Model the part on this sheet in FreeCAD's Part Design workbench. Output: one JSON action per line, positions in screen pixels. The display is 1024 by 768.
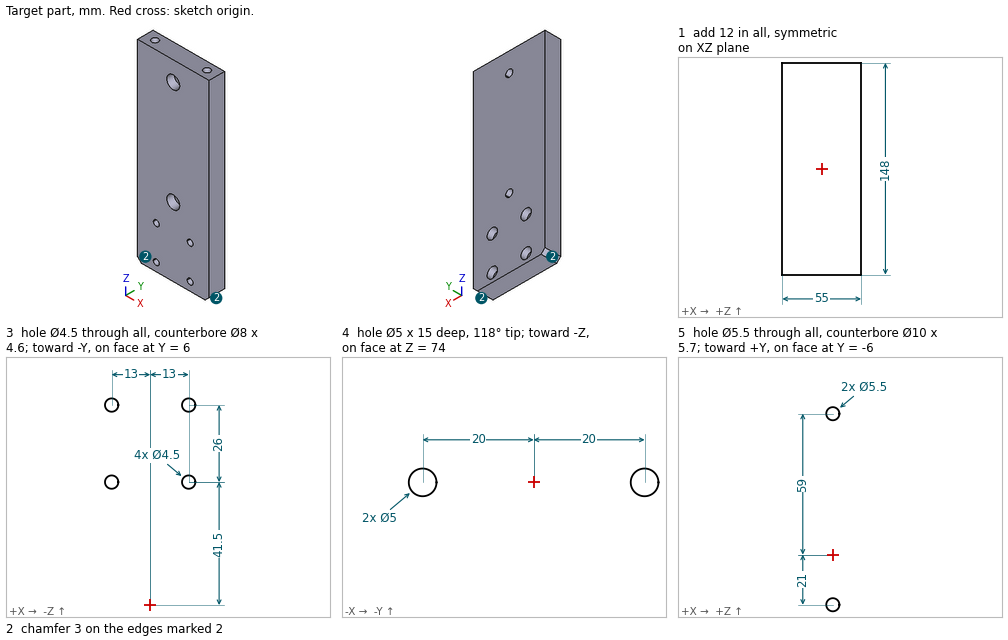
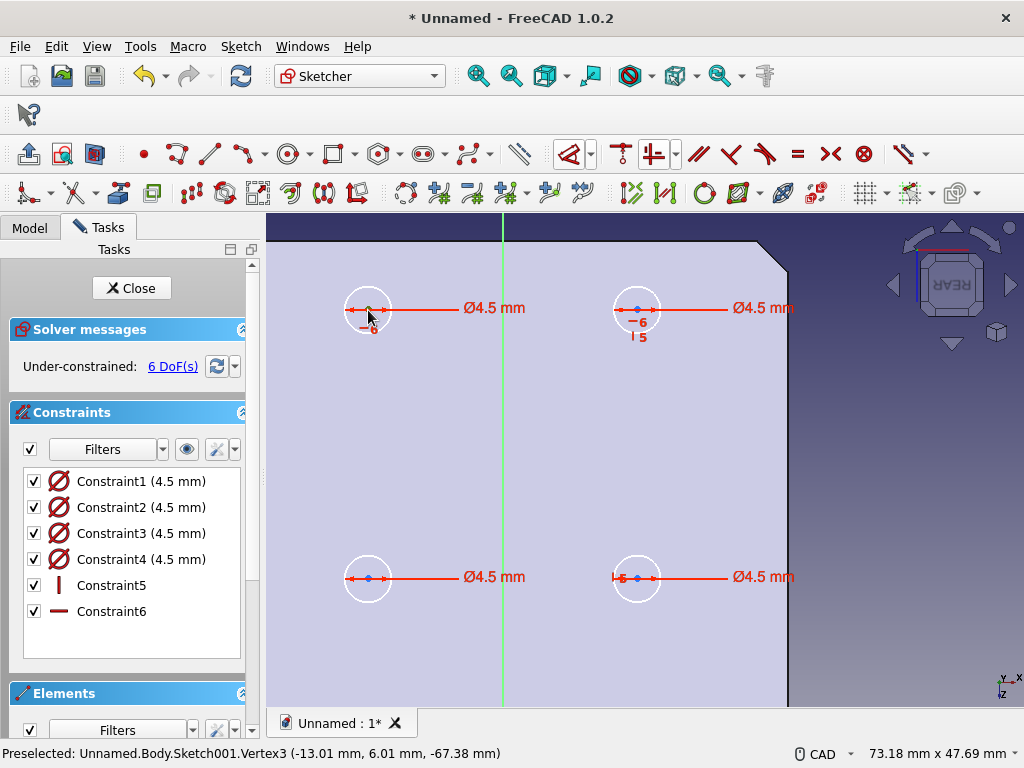
{"action": "left_click", "coordinate": [368, 579]}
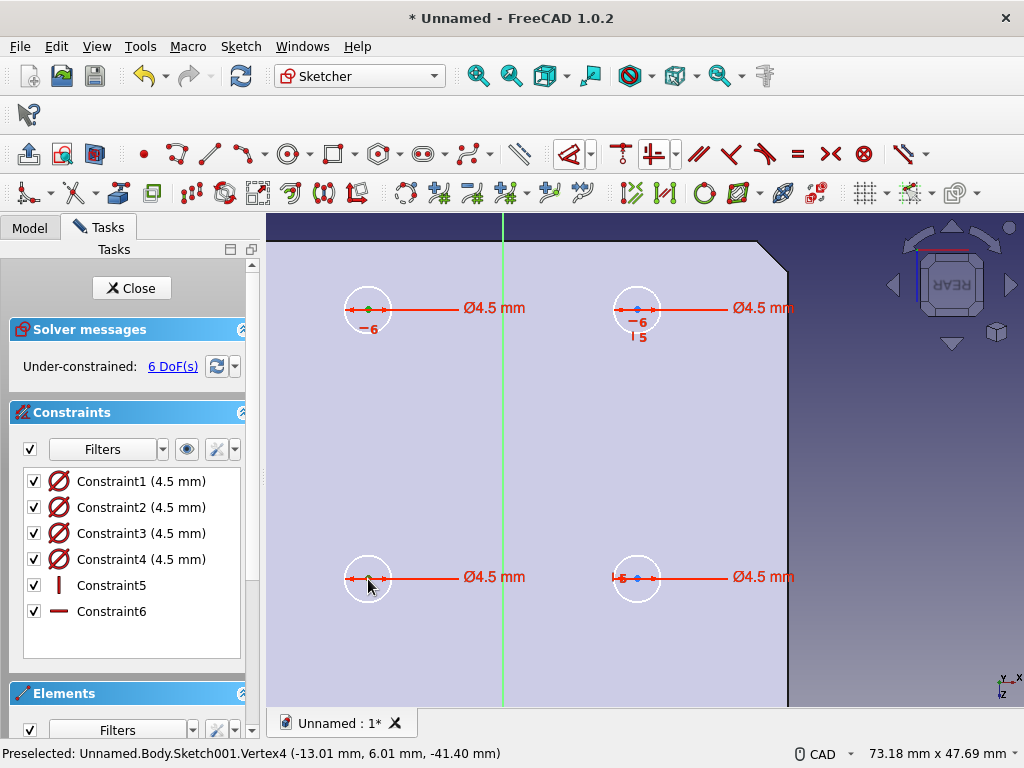
{"action": "key", "text": "v"}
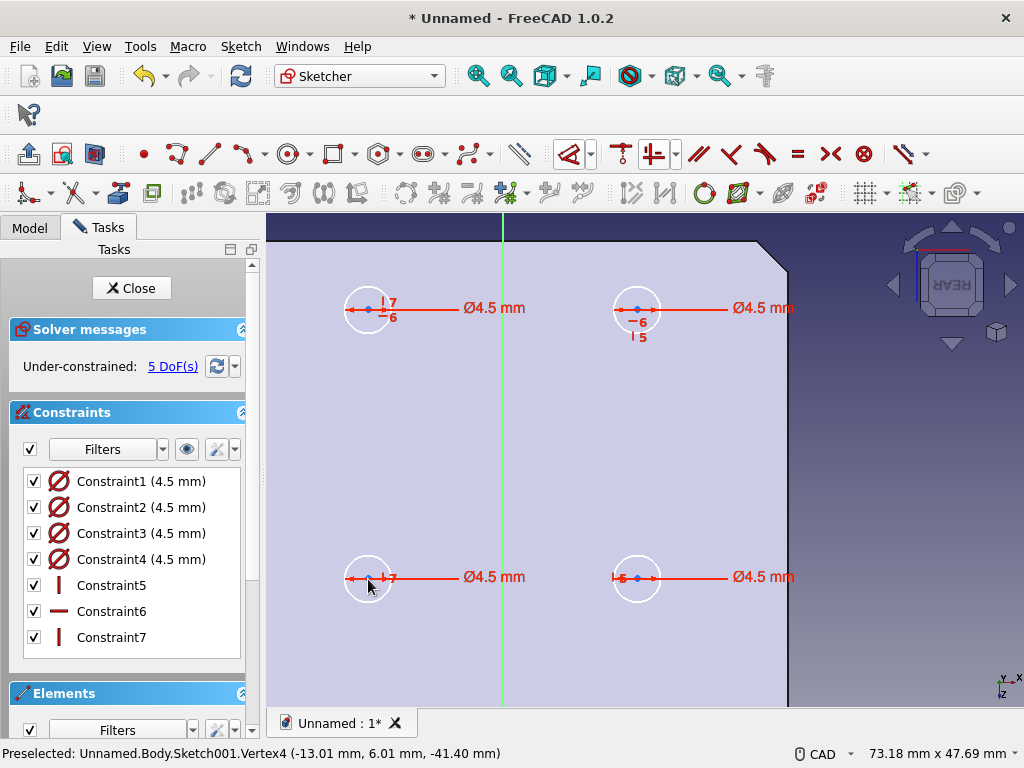
{"action": "left_click", "coordinate": [637, 579]}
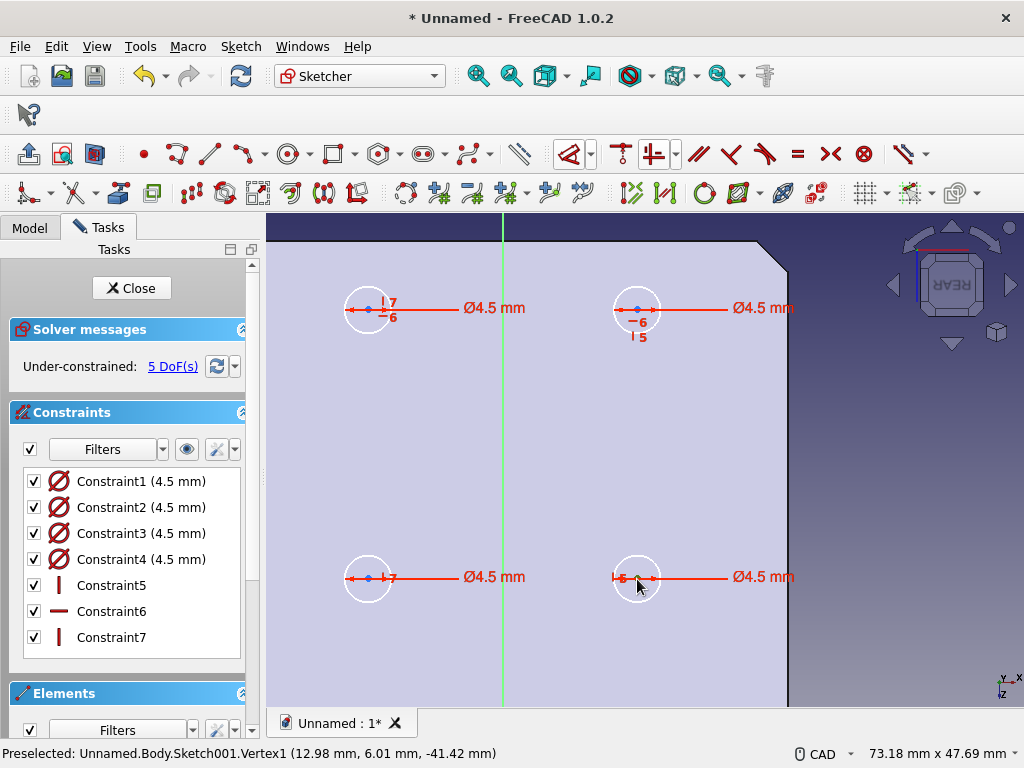
{"action": "left_click", "coordinate": [368, 579]}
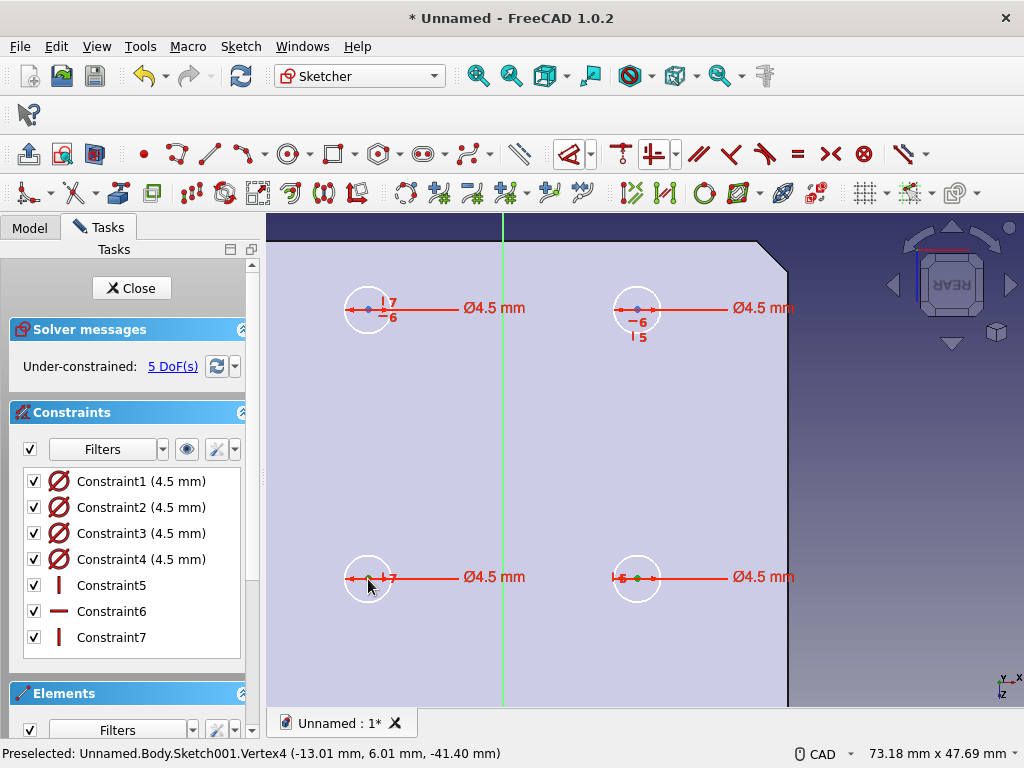
{"action": "left_click", "coordinate": [676, 154]}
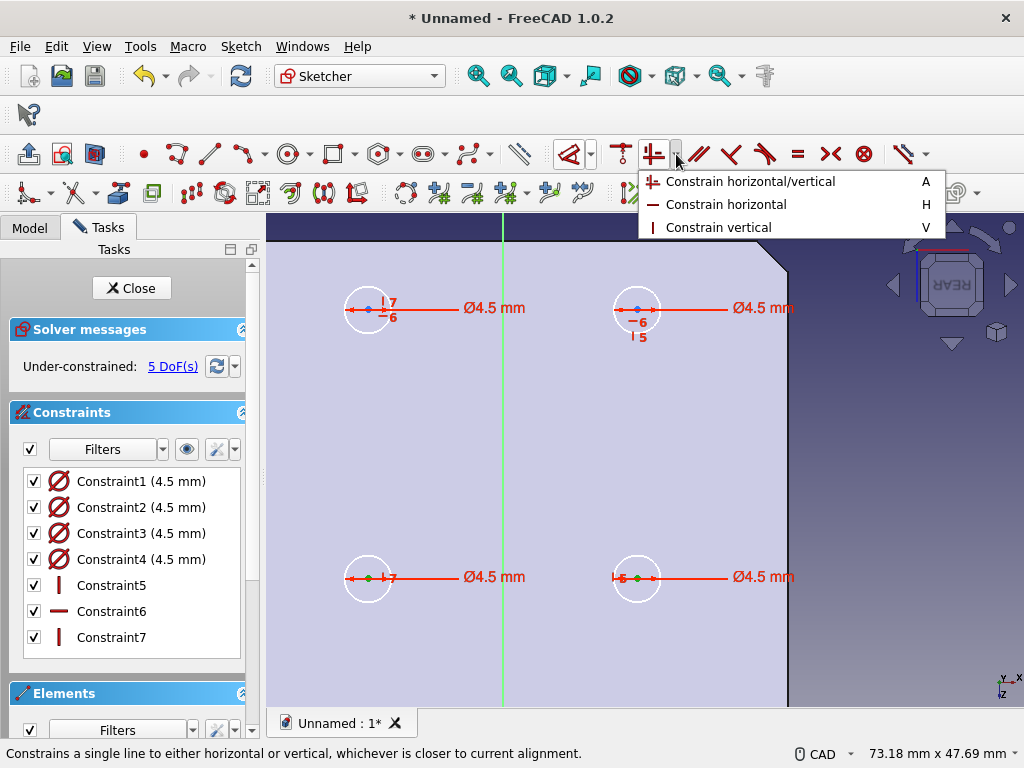
{"action": "left_click", "coordinate": [792, 204]}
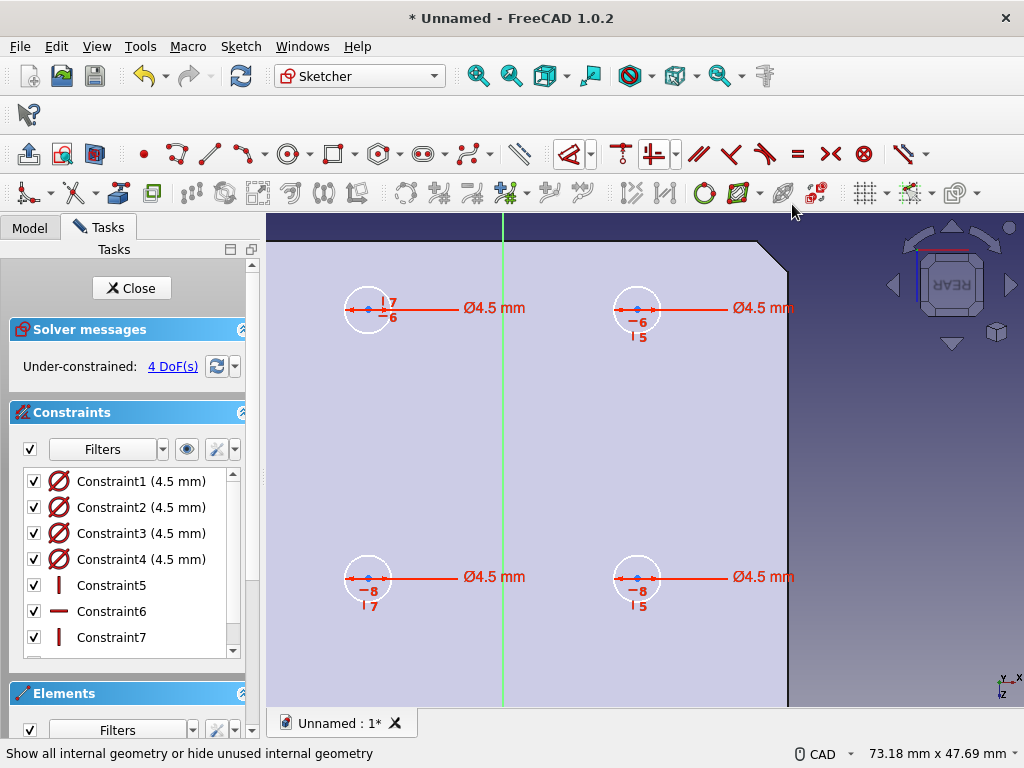
{"action": "left_click", "coordinate": [568, 154]}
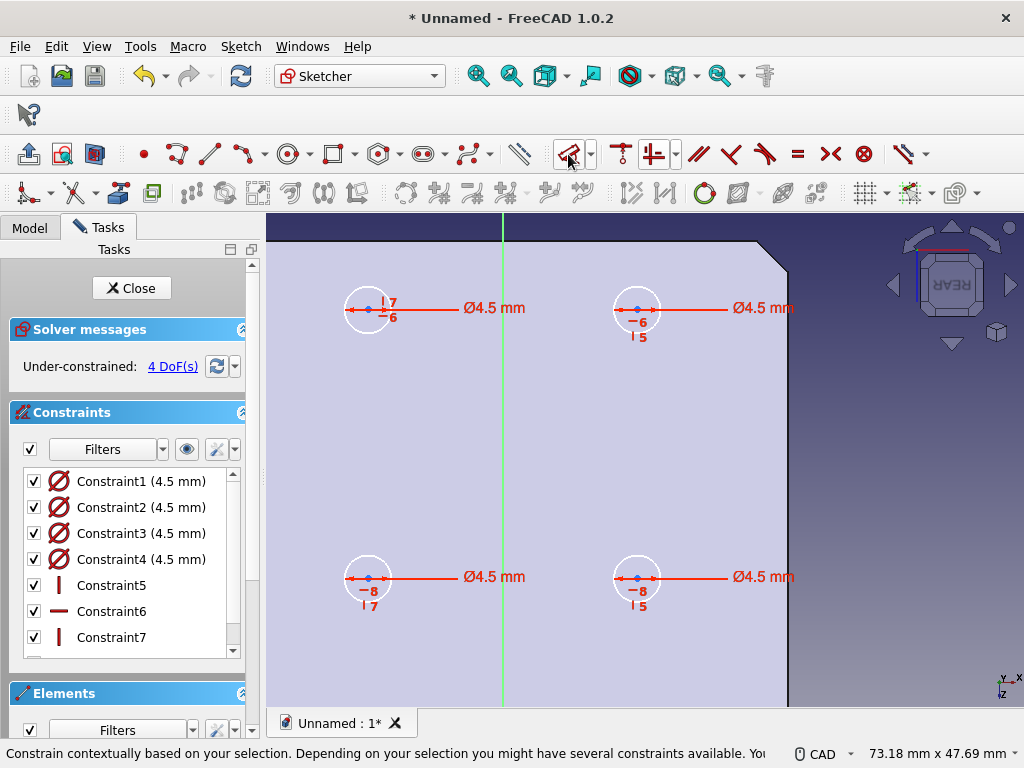
{"action": "left_click", "coordinate": [637, 579]}
{"action": "left_click", "coordinate": [570, 545]}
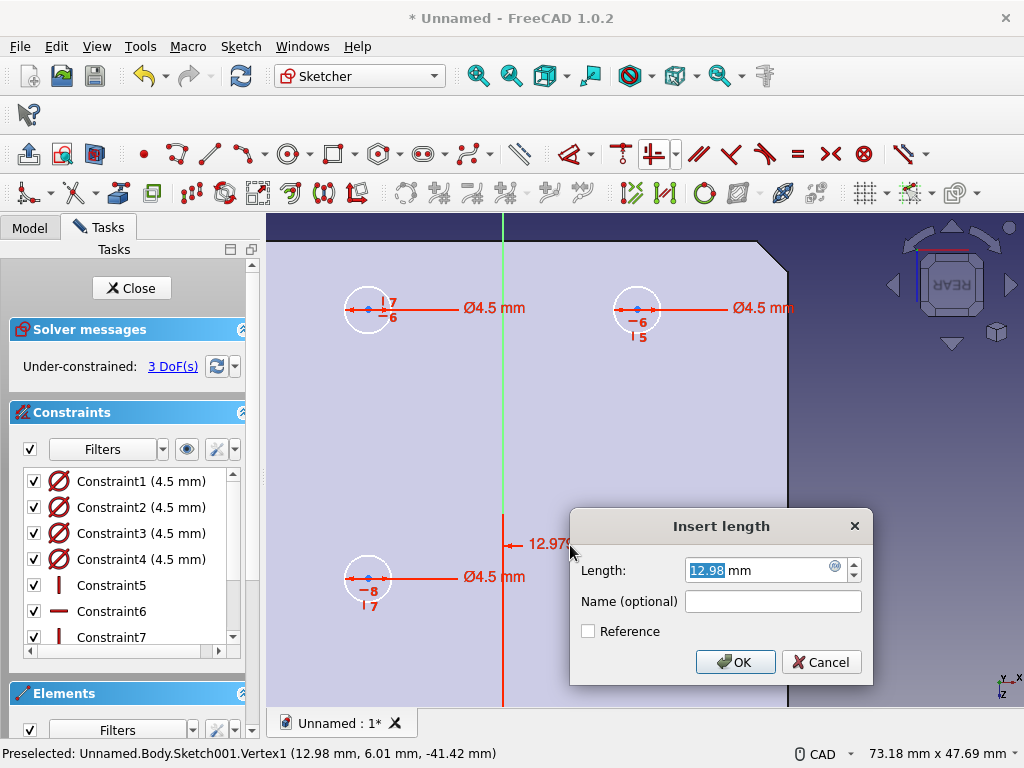
{"action": "type", "text": "13"}
{"action": "key", "text": "Return"}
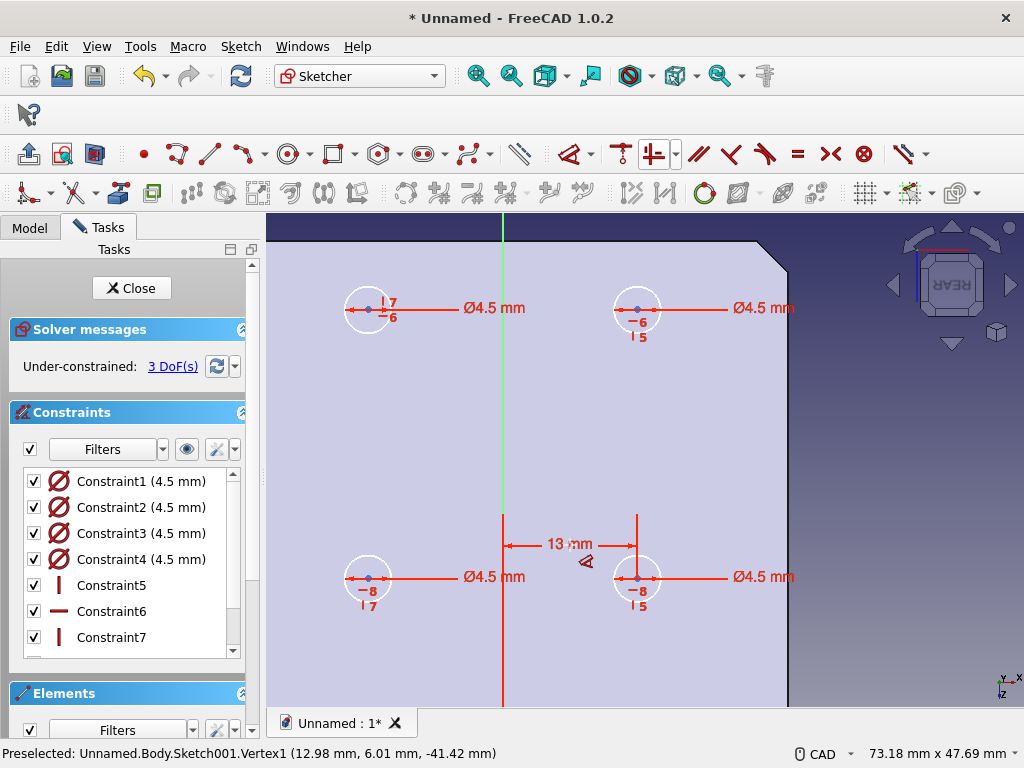
{"action": "left_click", "coordinate": [368, 310]}
{"action": "left_click", "coordinate": [435, 276]}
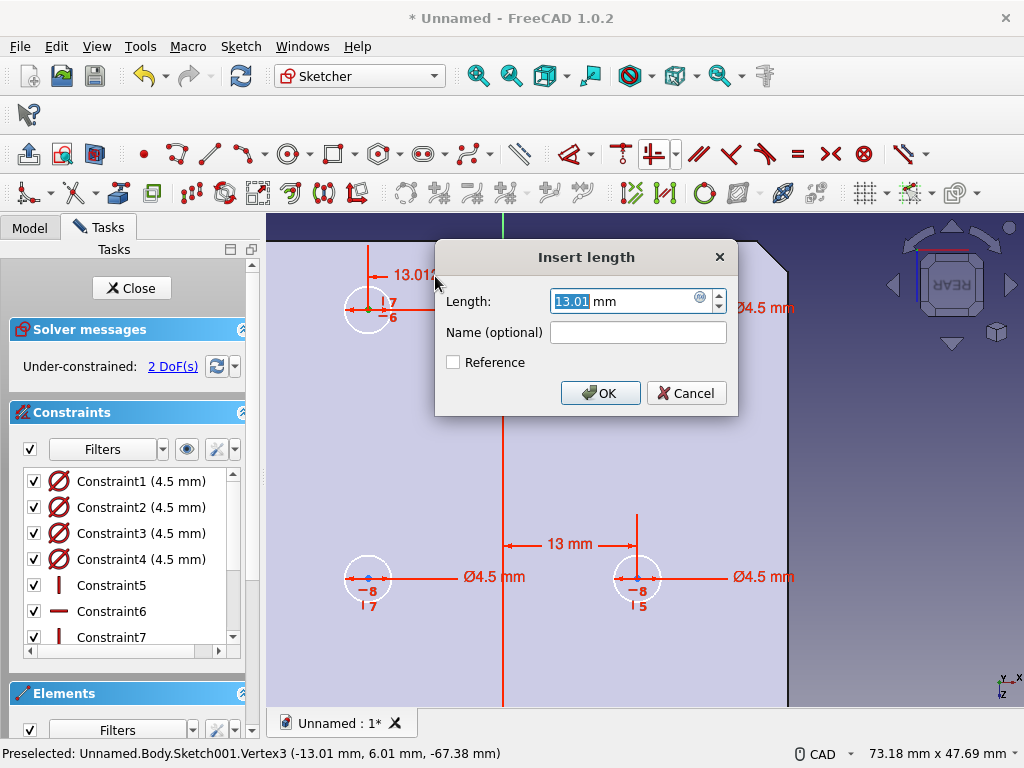
{"action": "type", "text": "13"}
{"action": "key", "text": "Return"}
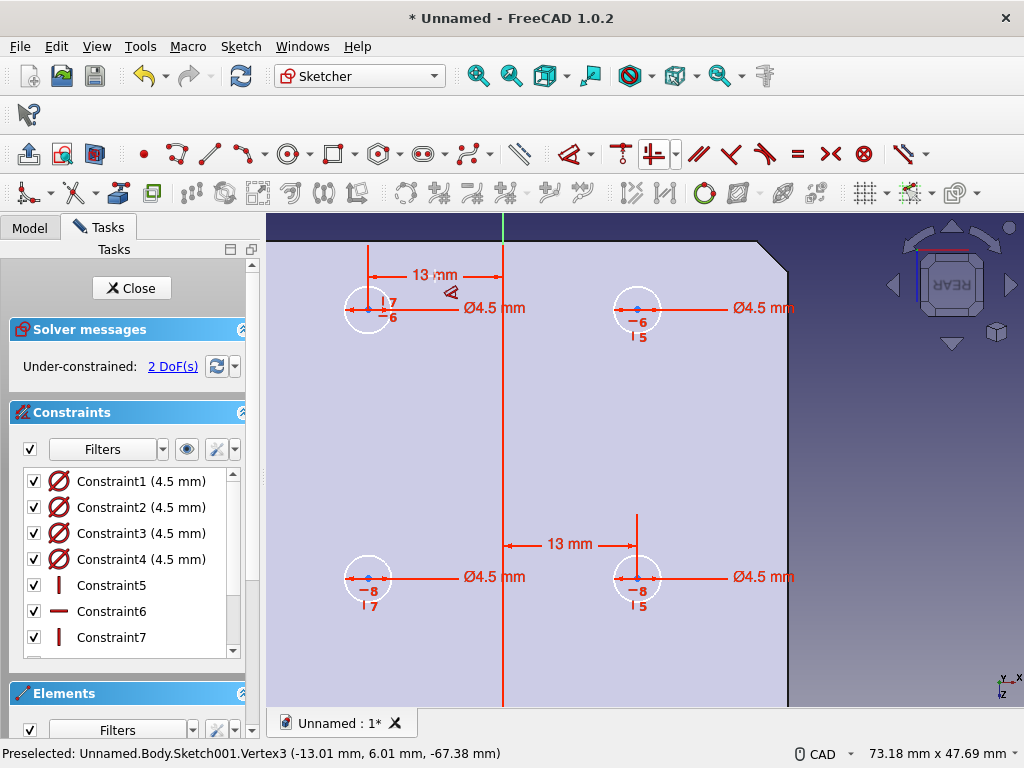
{"action": "left_click", "coordinate": [637, 579]}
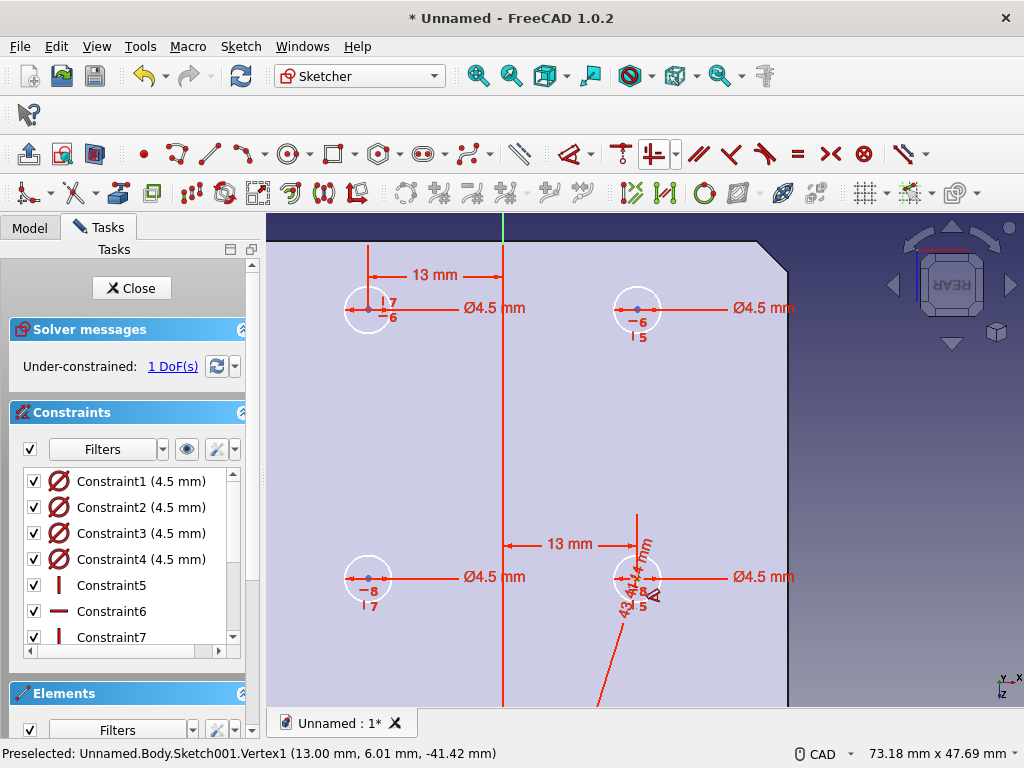
{"action": "left_click", "coordinate": [637, 310]}
{"action": "left_click", "coordinate": [671, 444]}